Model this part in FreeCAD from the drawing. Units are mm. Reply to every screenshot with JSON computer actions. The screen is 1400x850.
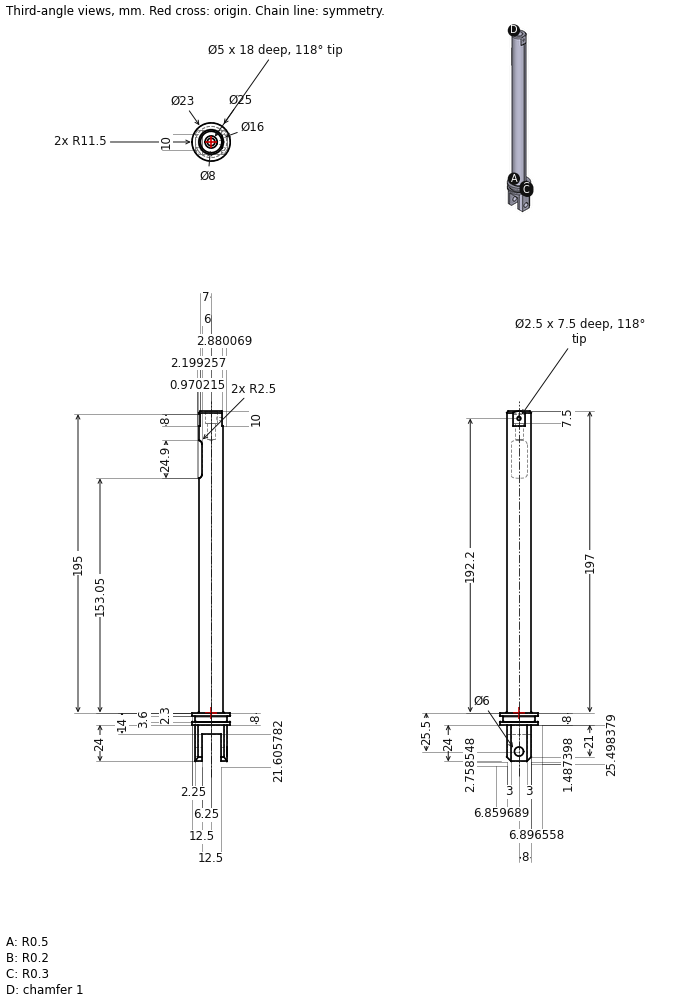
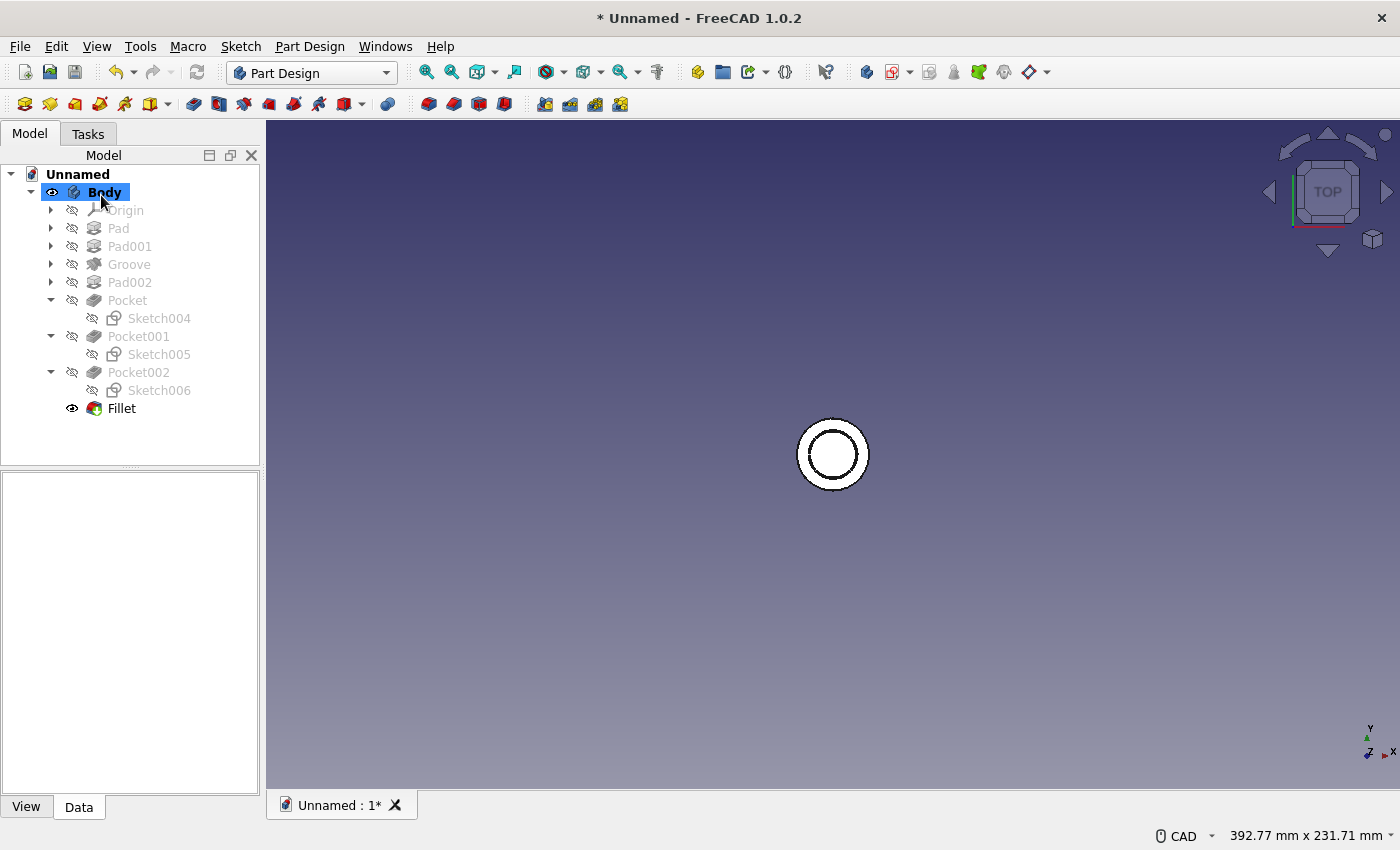
{"action": "left_click", "coordinate": [427, 72]}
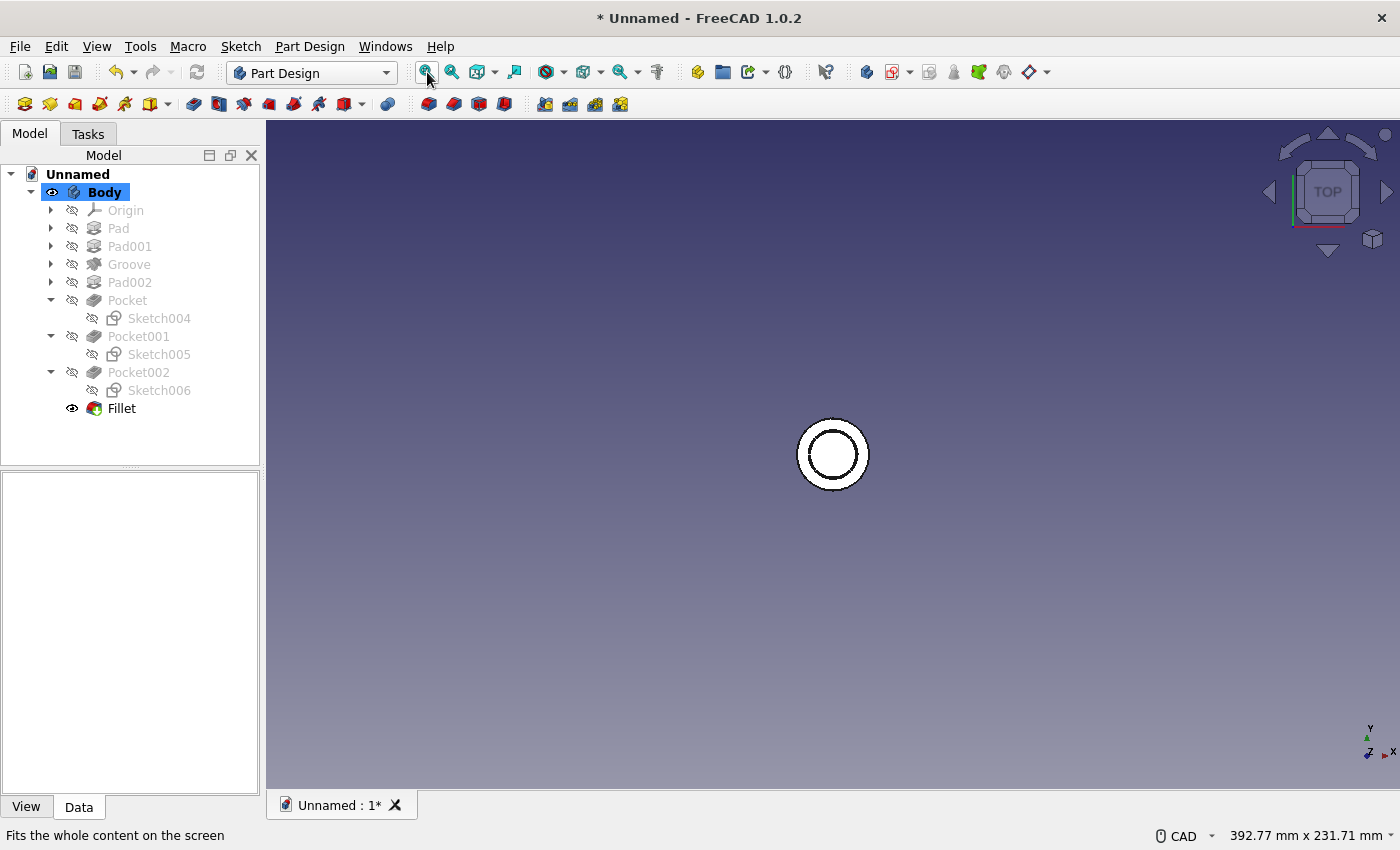
{"action": "key", "text": "0"}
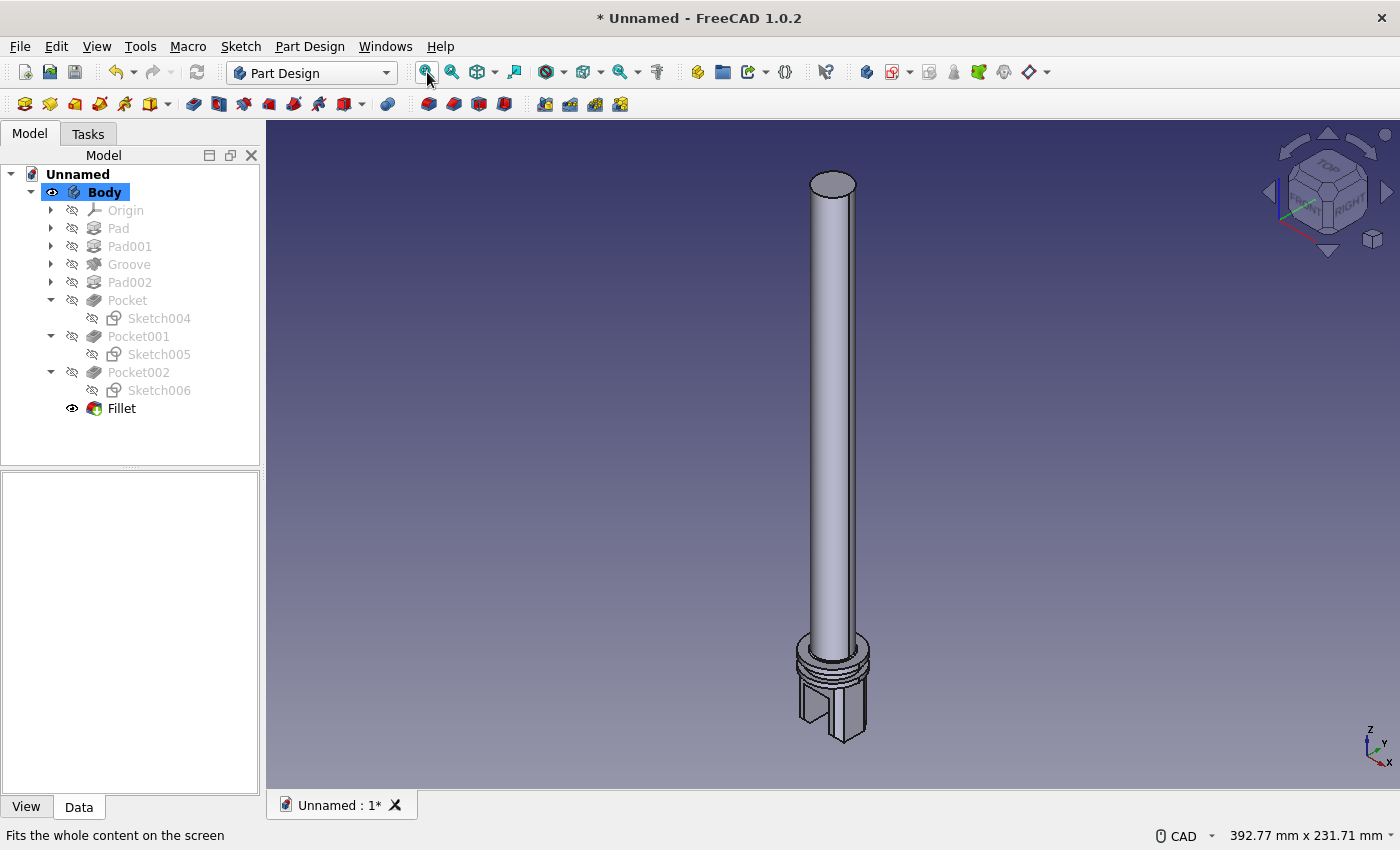
{"action": "key", "text": "1"}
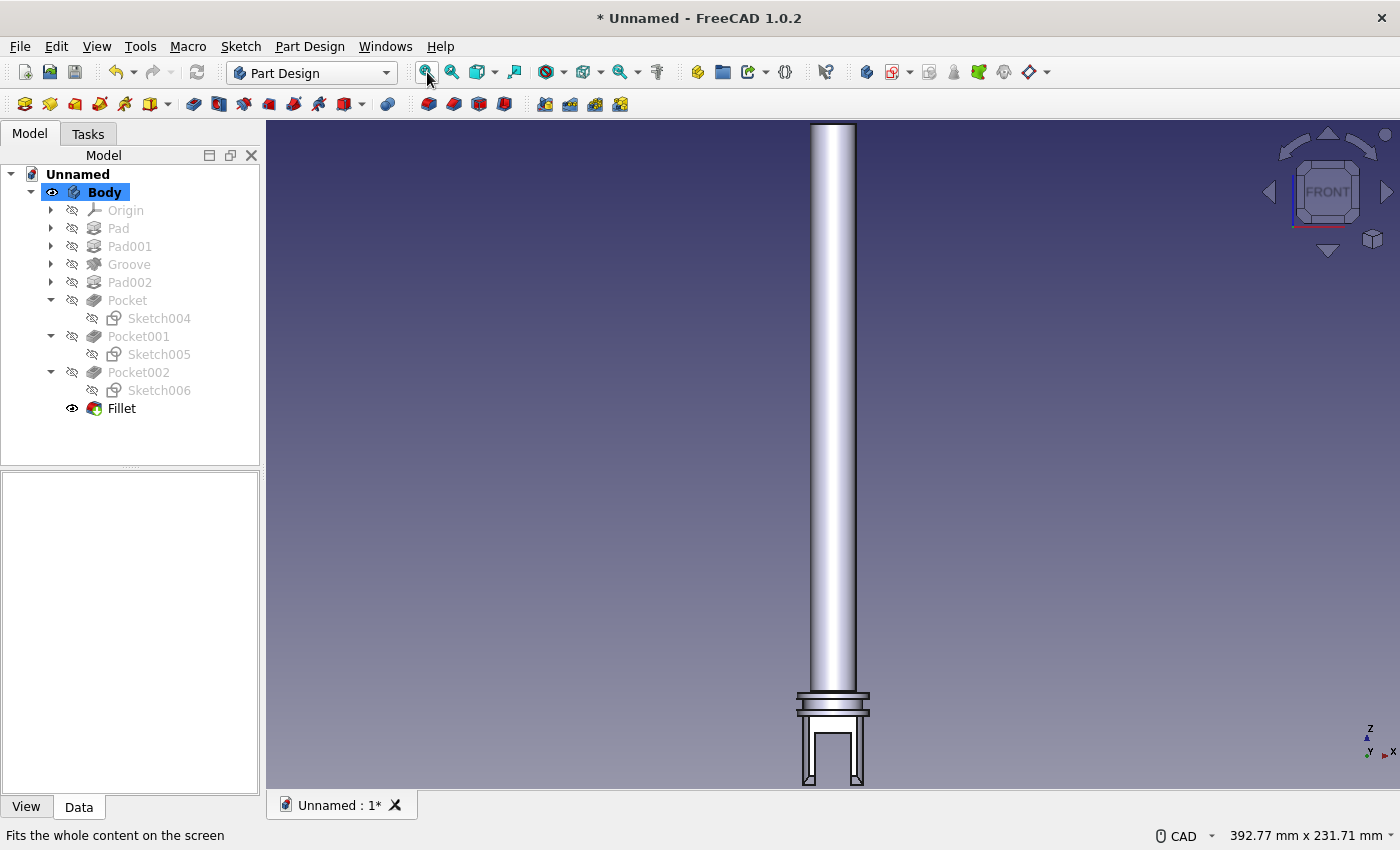
{"action": "key", "text": "3"}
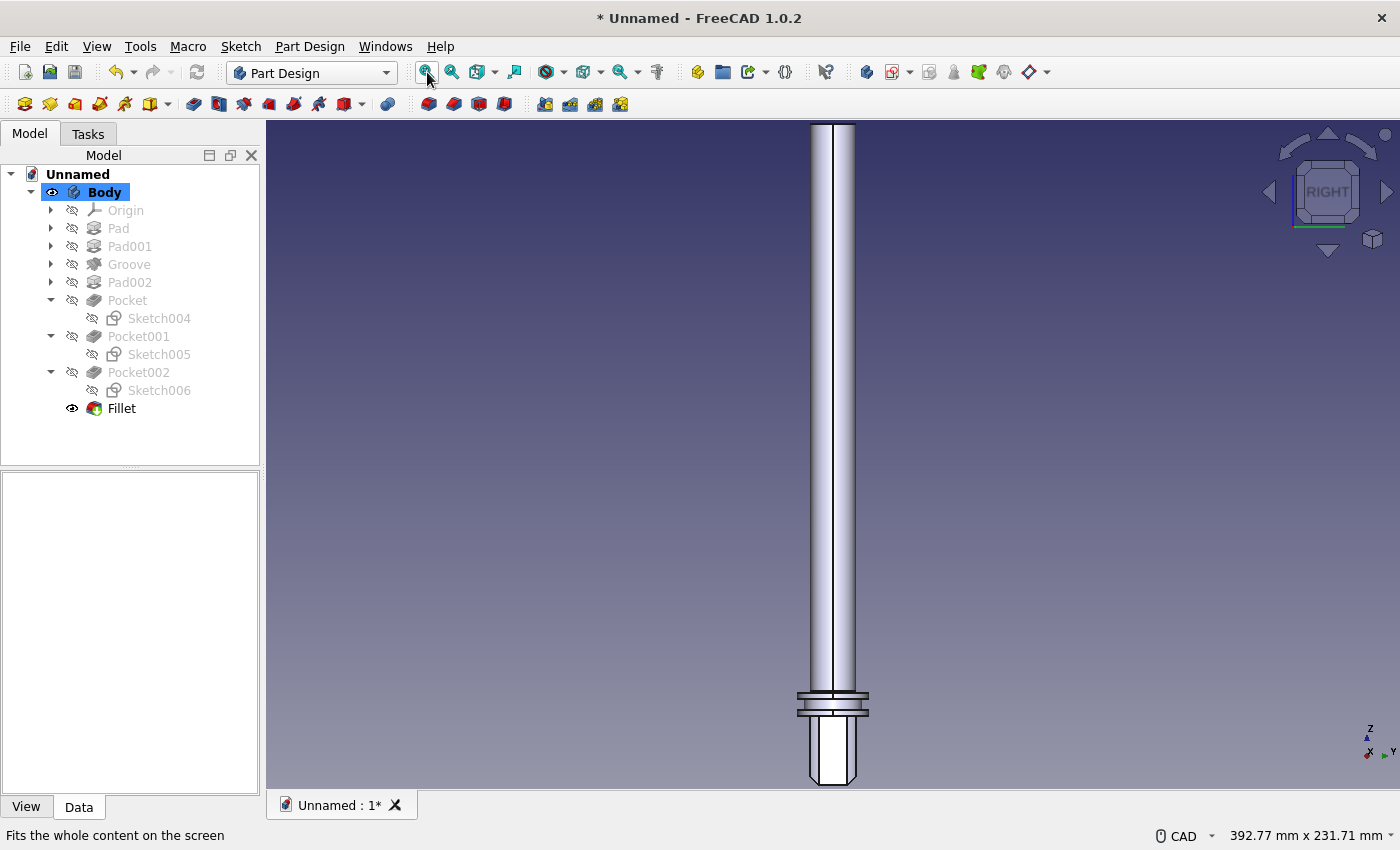
{"action": "left_click", "coordinate": [867, 698]}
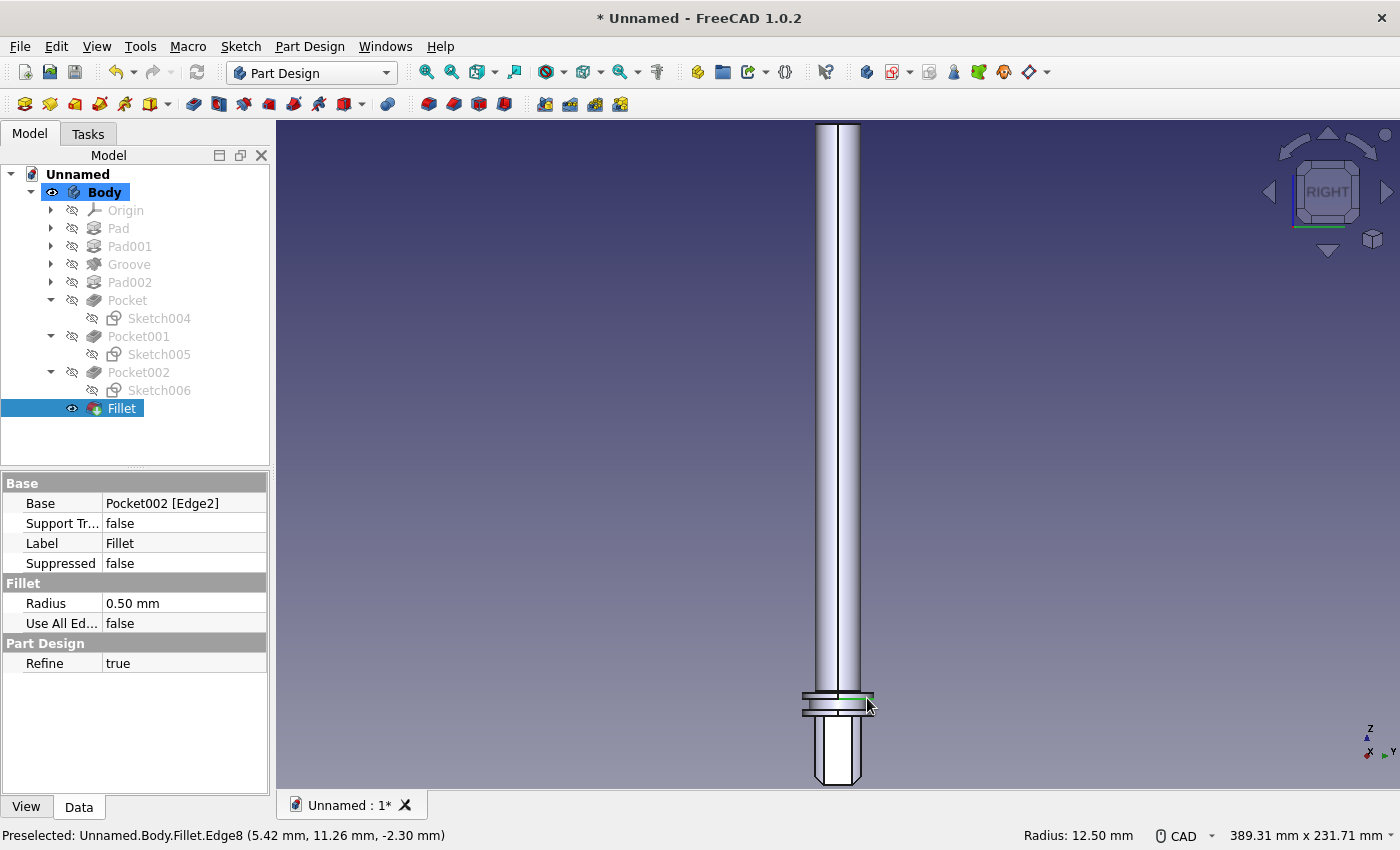
{"action": "left_click", "coordinate": [872, 709], "text": "ctrl"}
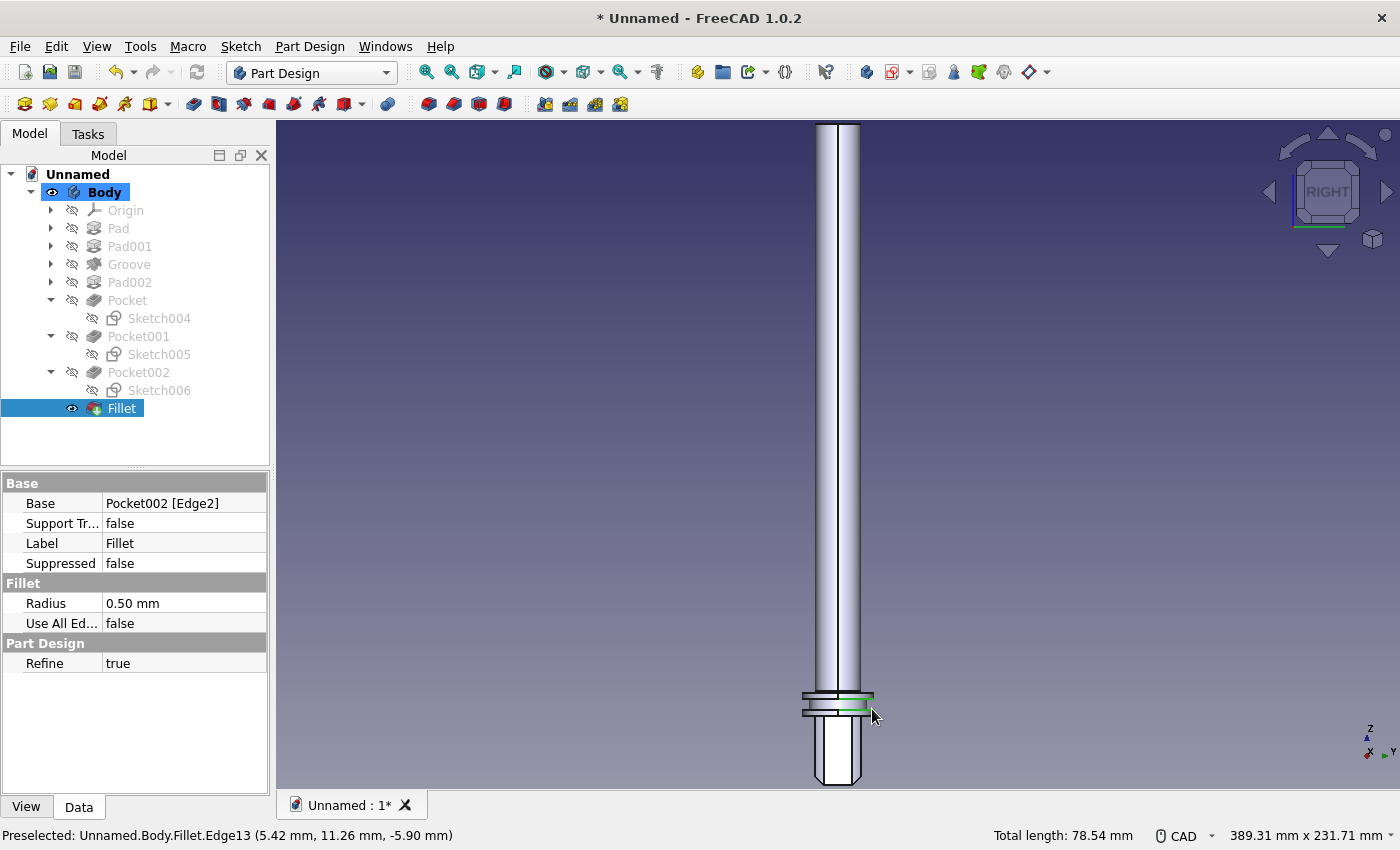
{"action": "left_click", "coordinate": [429, 104]}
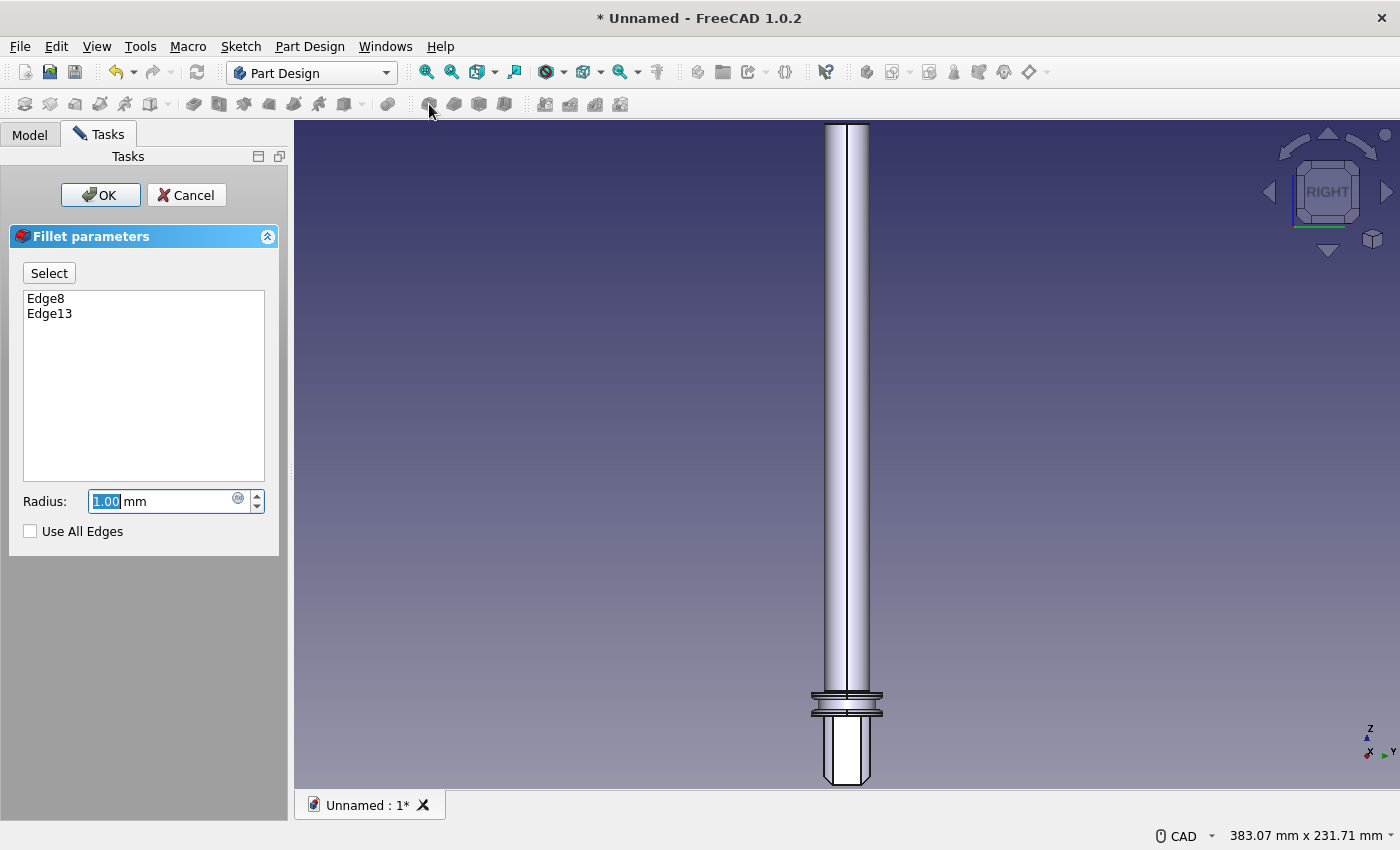
{"action": "type", "text": "0.2"}
{"action": "key", "text": "Tab"}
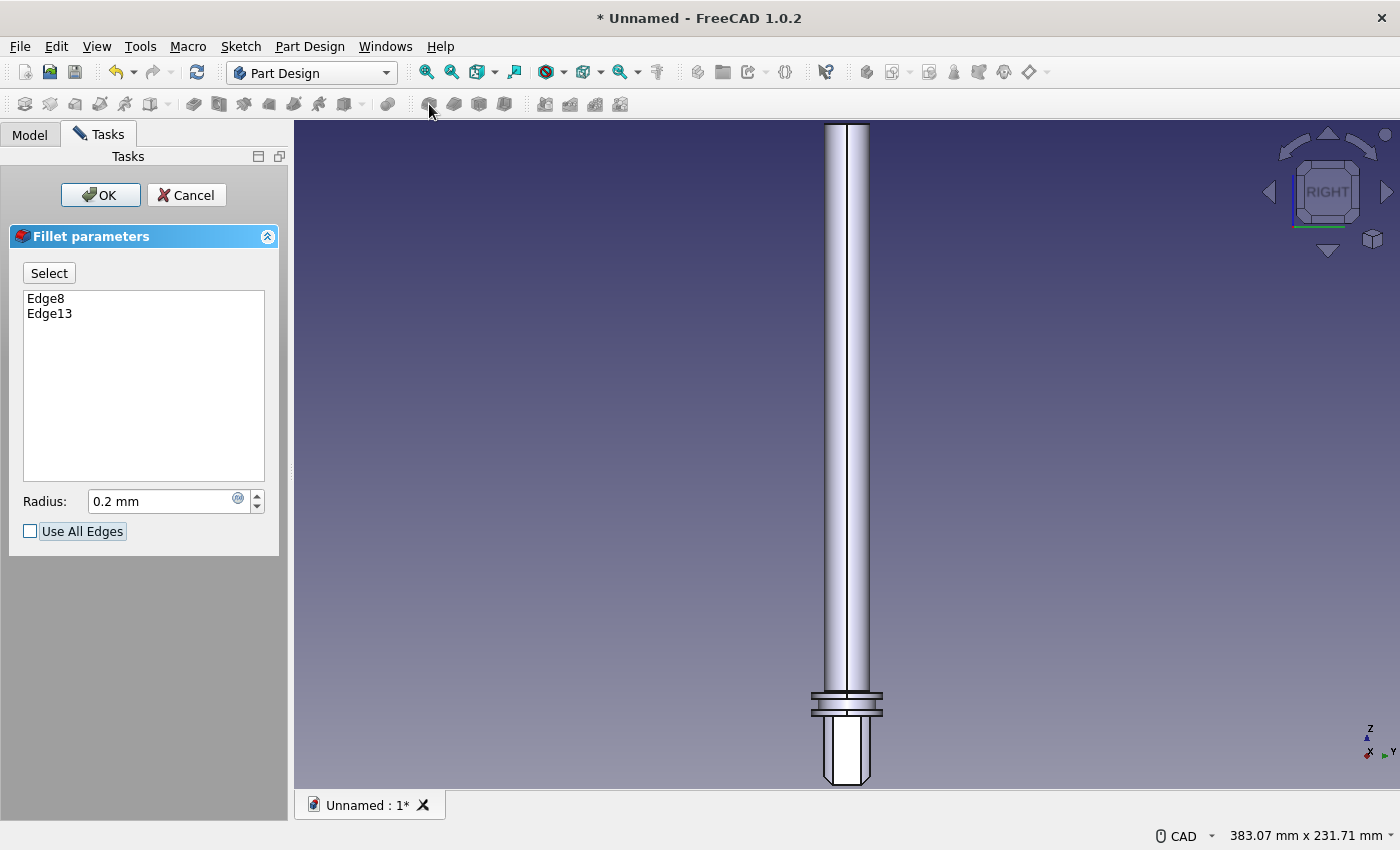
{"action": "left_click", "coordinate": [101, 195]}